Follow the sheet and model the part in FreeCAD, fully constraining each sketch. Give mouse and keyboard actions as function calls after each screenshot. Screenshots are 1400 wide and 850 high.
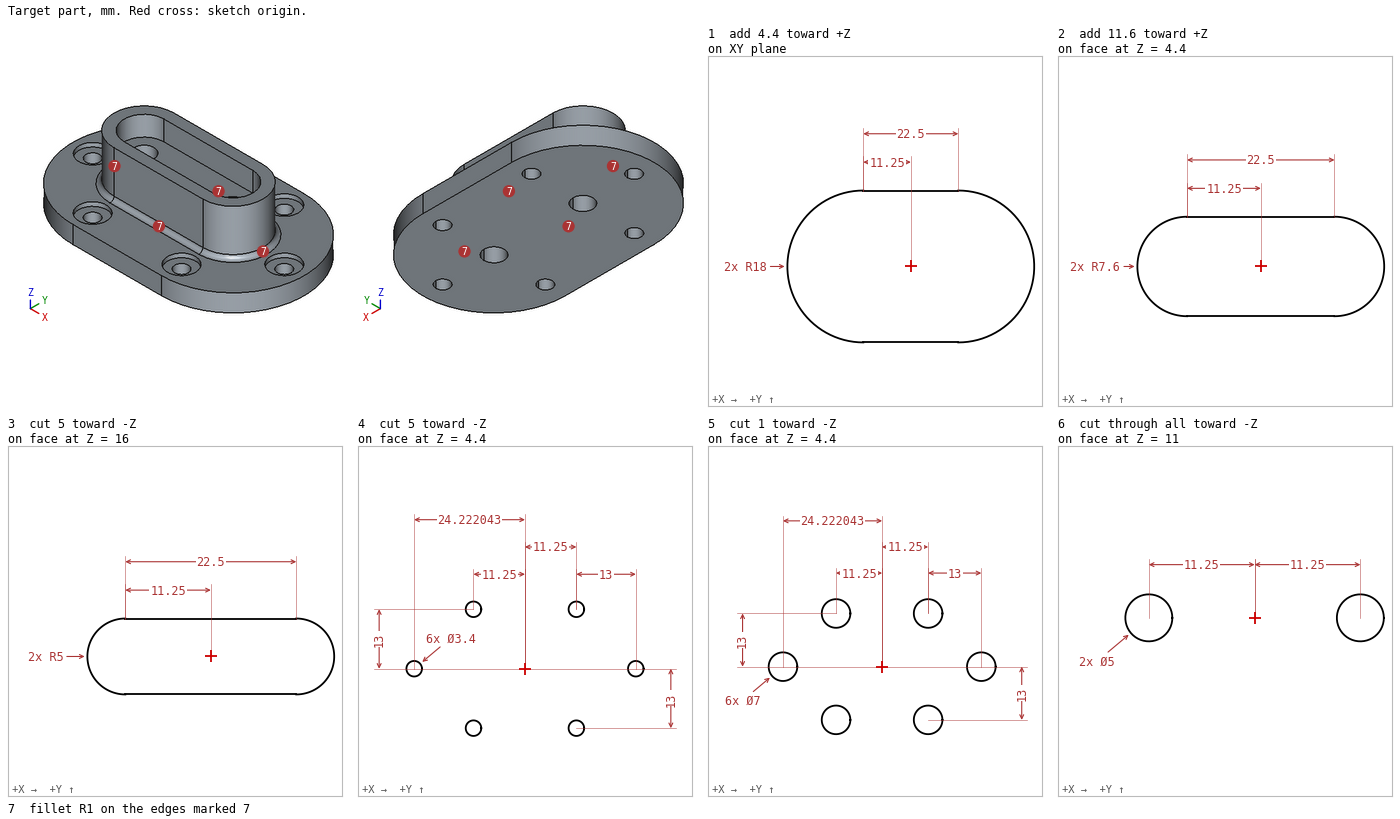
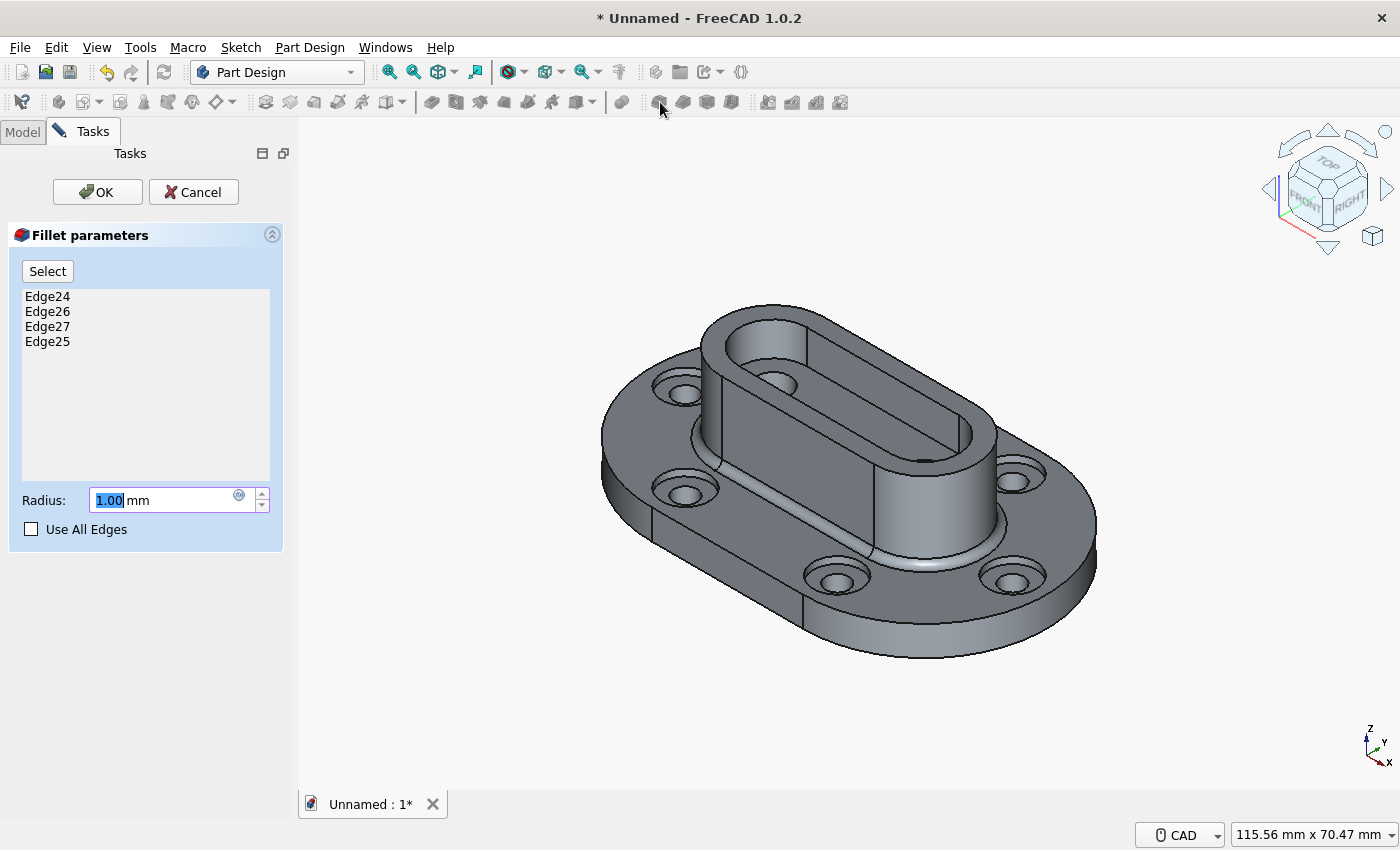
text(1)
key(Tab)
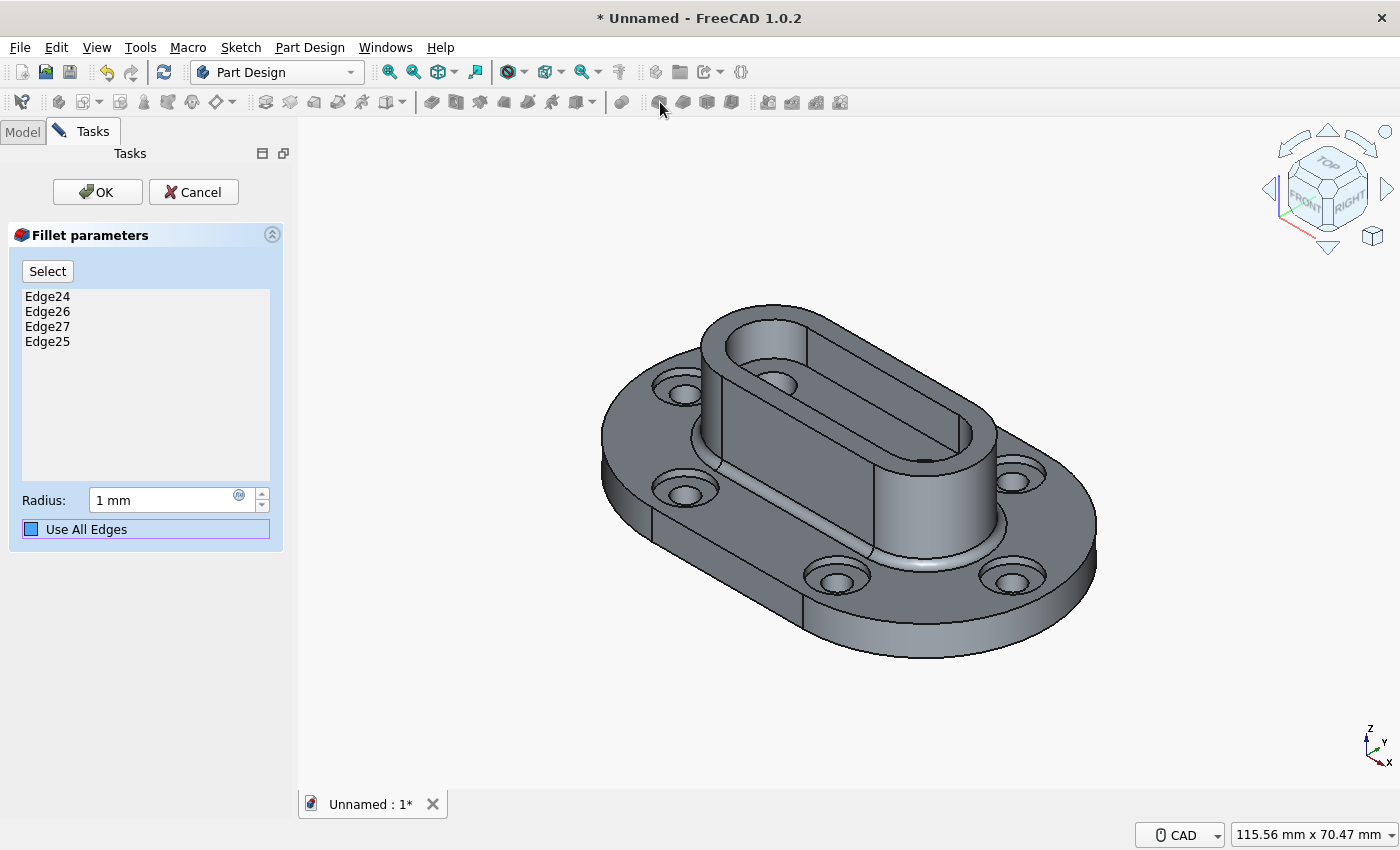
click(98, 192)